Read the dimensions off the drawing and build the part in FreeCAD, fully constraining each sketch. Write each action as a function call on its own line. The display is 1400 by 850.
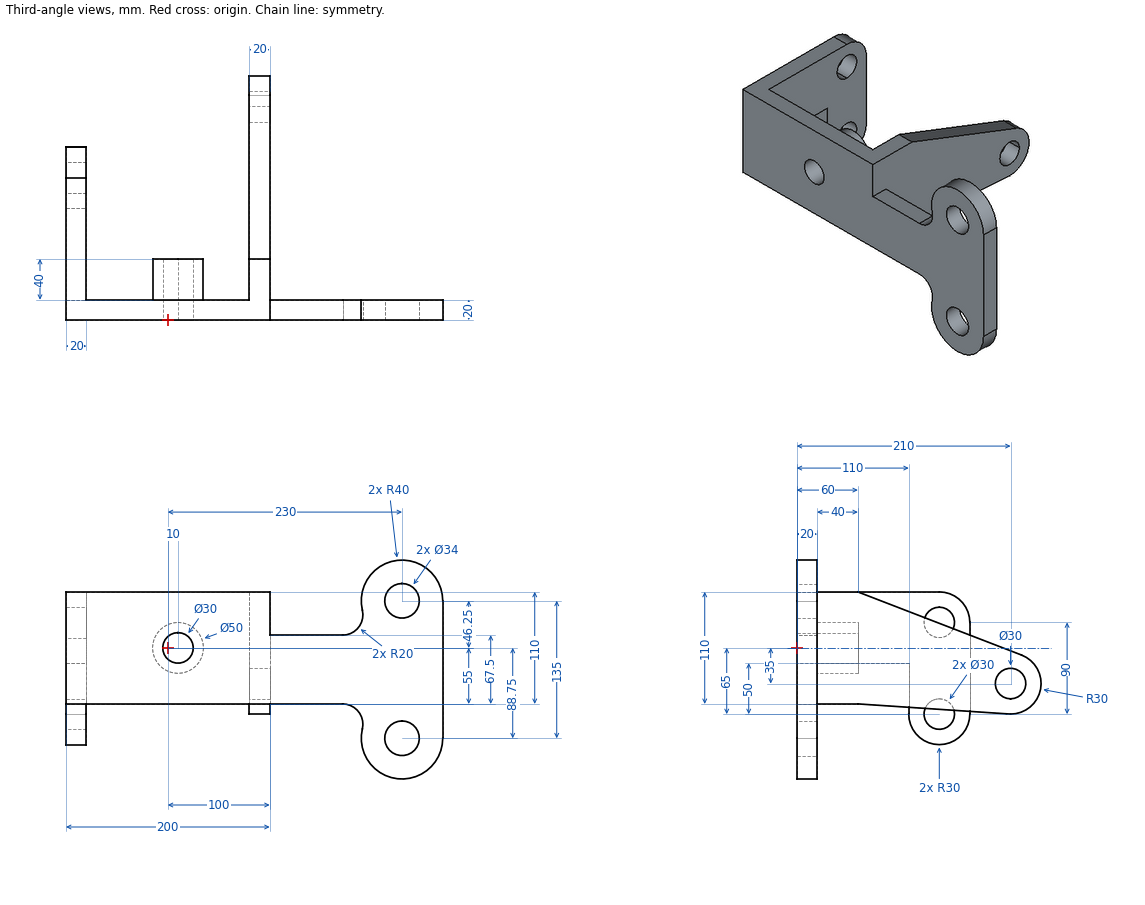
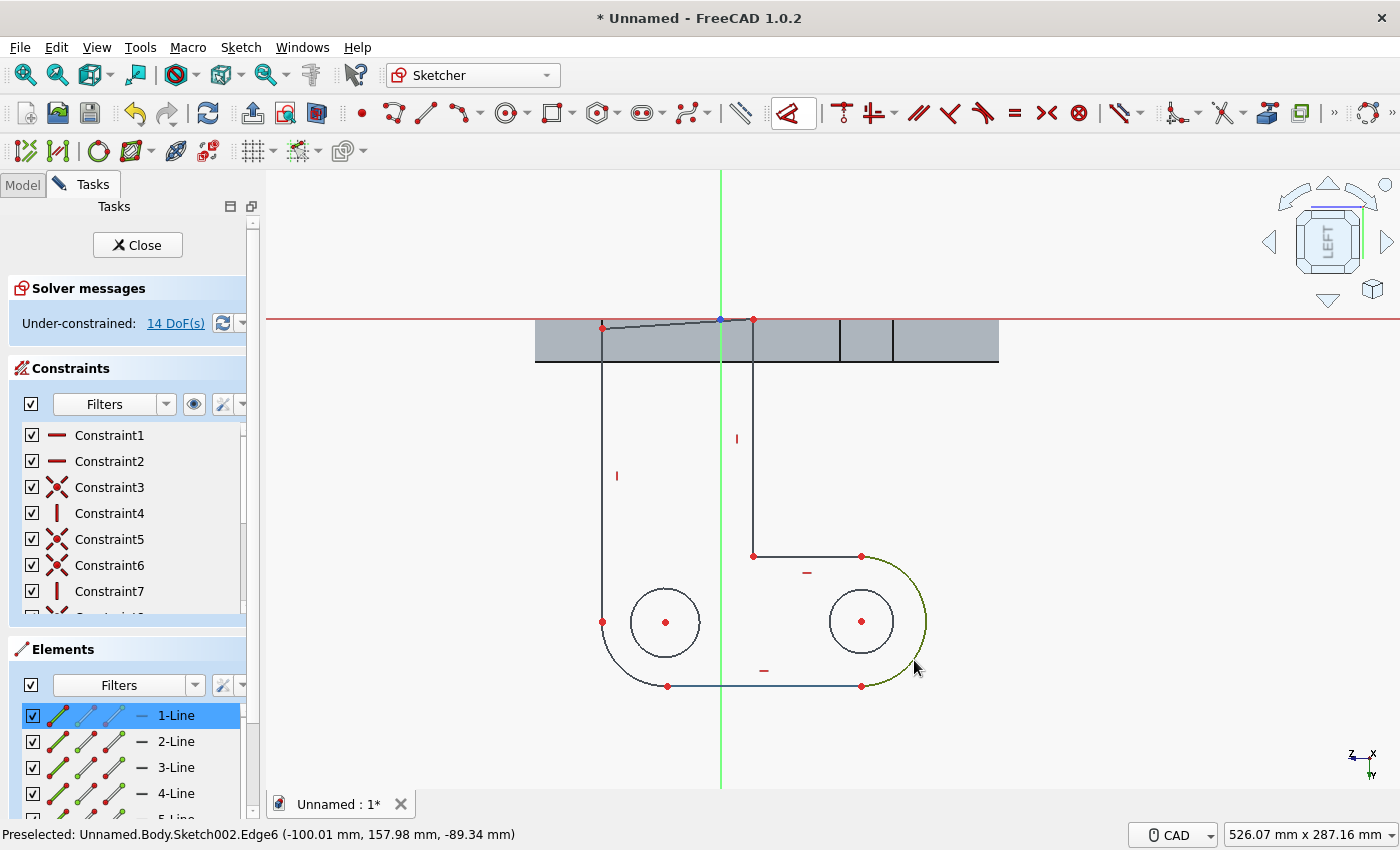
key(t)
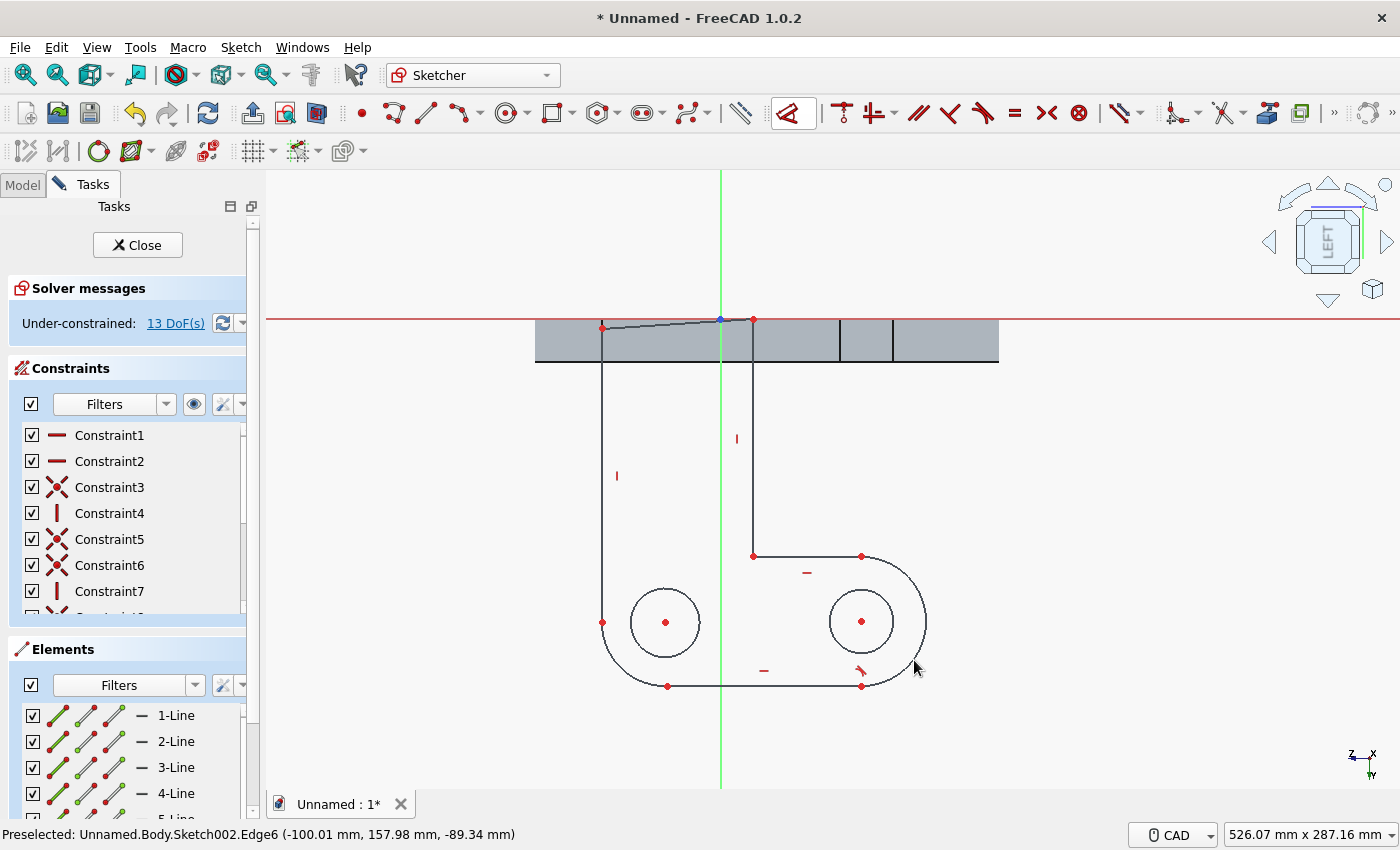
click(803, 686)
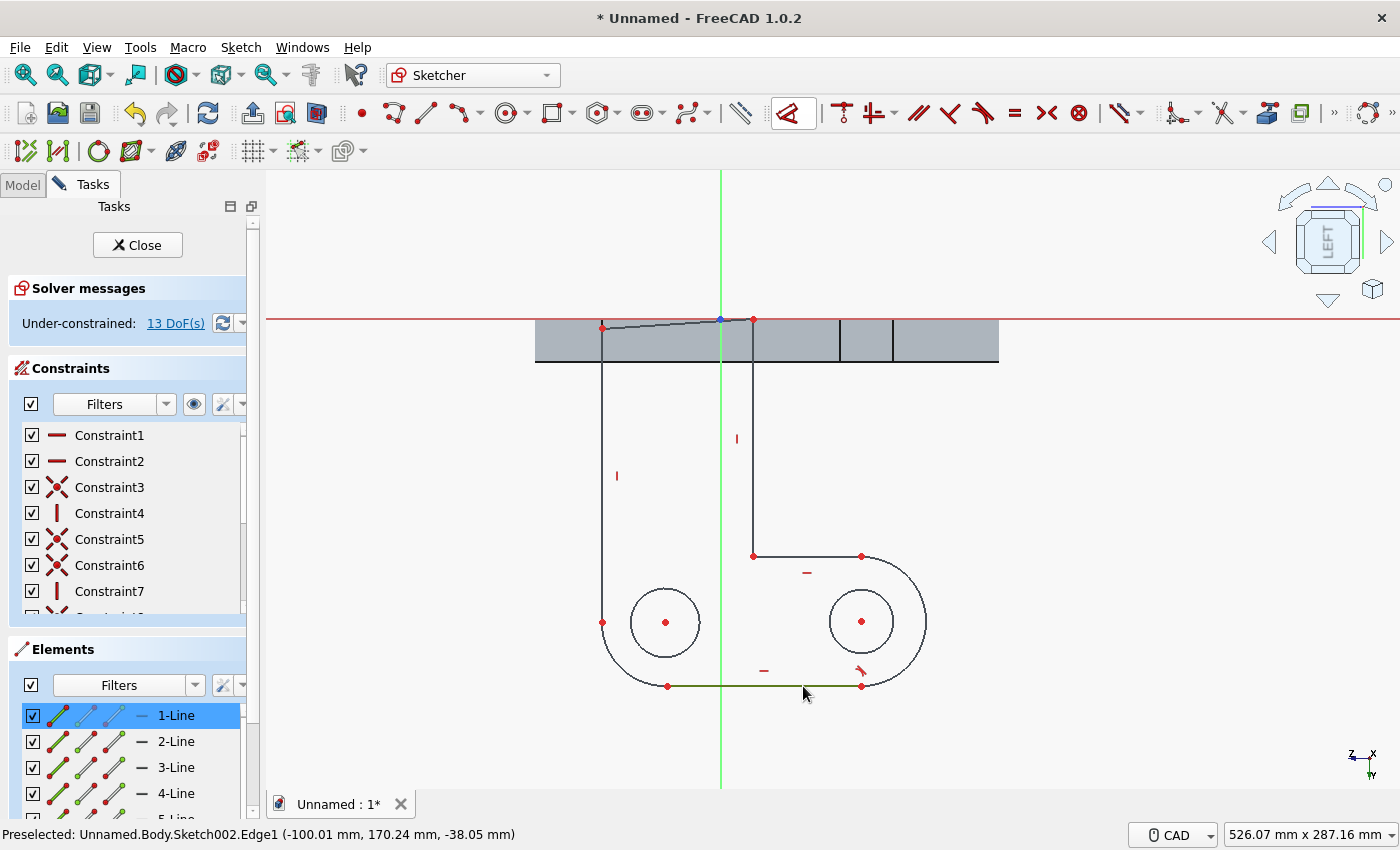
click(609, 651)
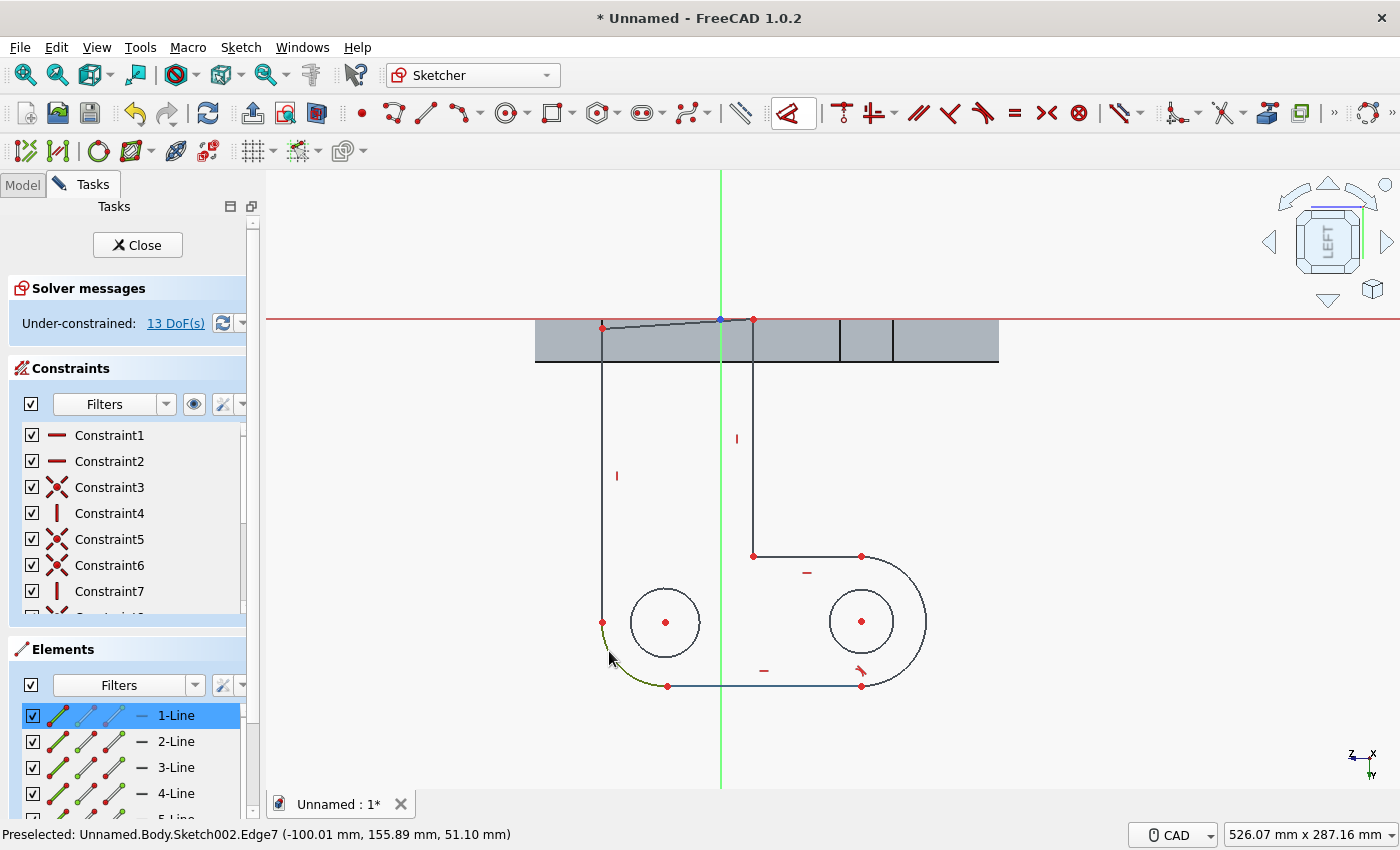
key(t)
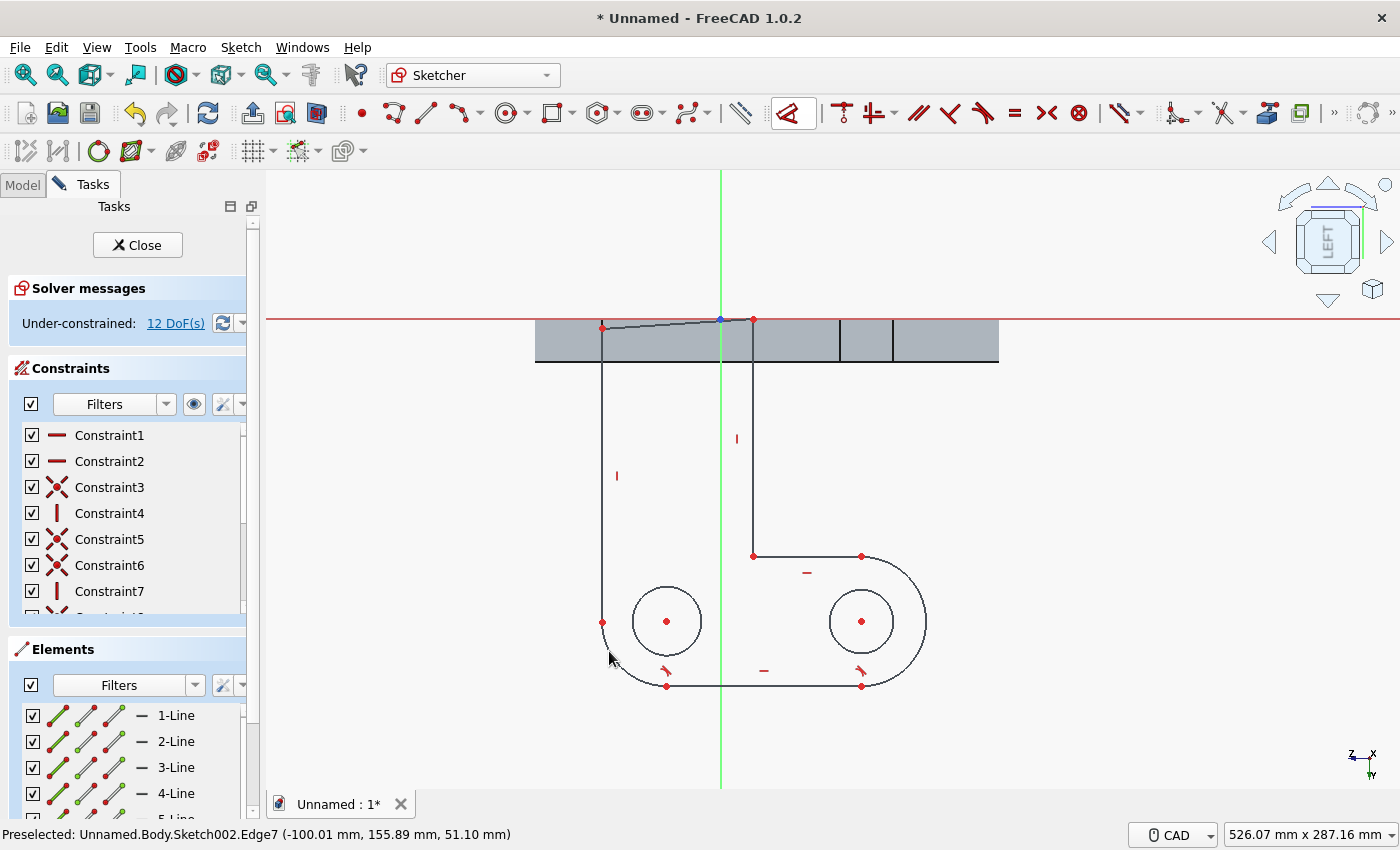
click(829, 557)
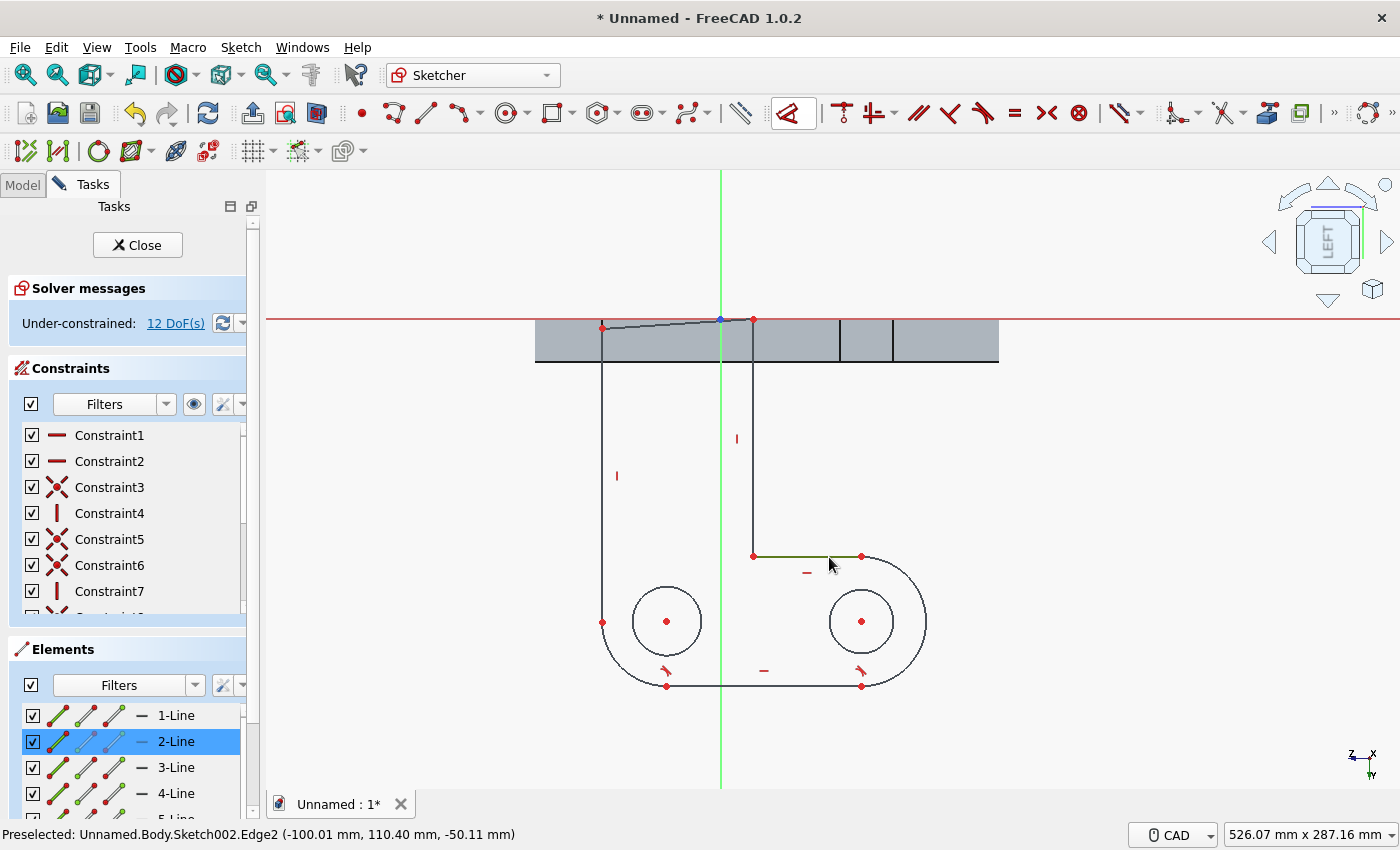
click(914, 659)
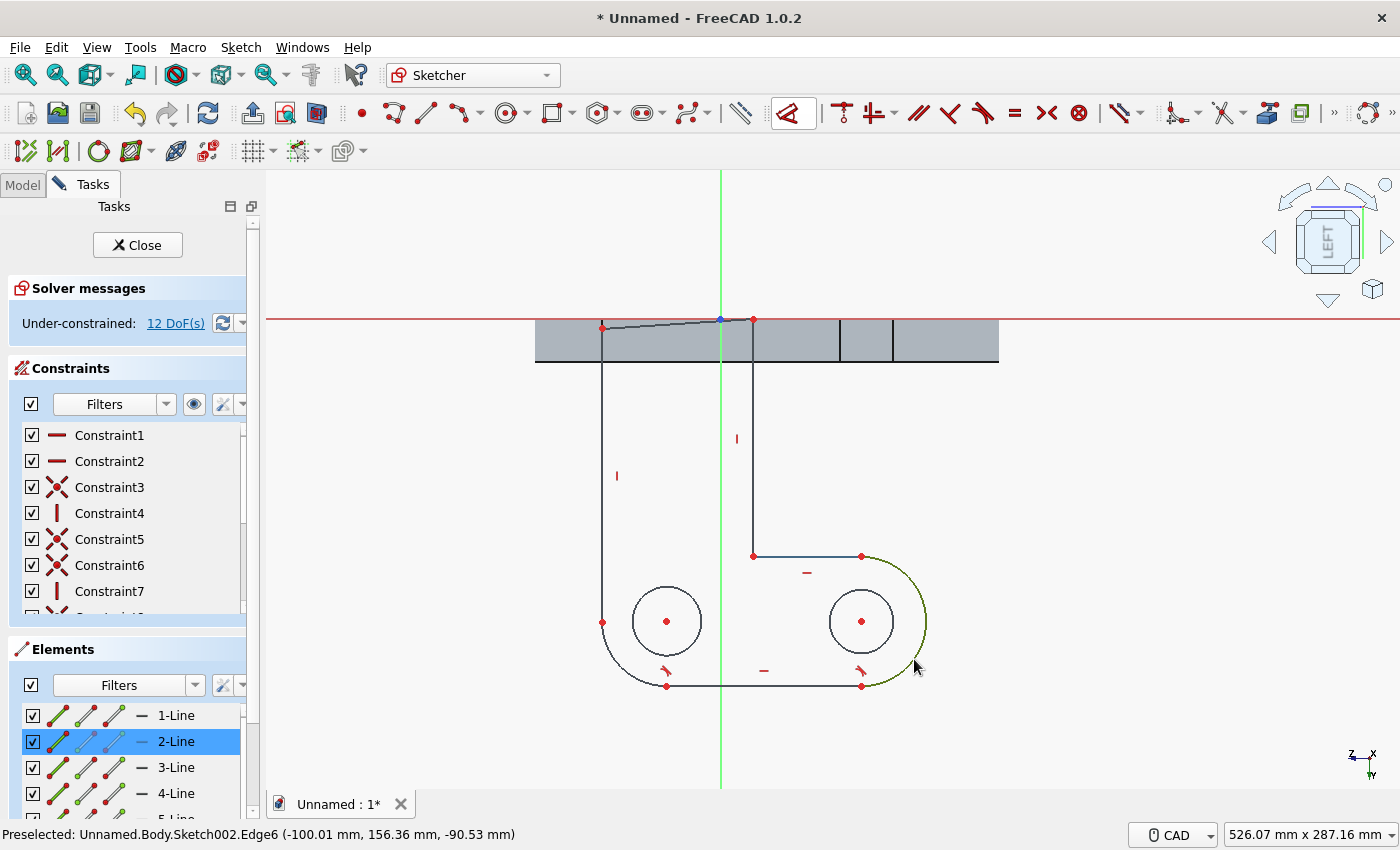
click(984, 114)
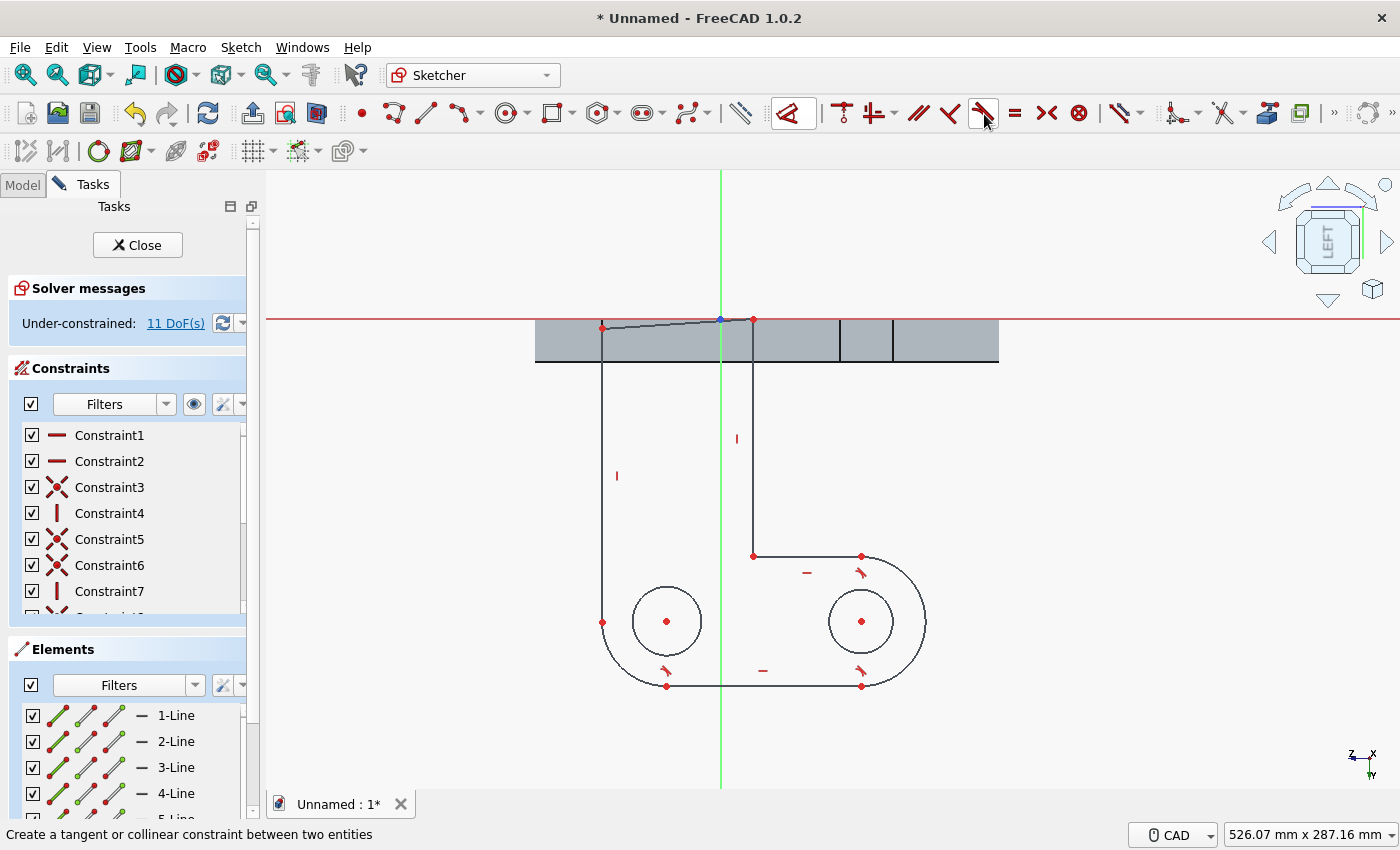
click(602, 417)